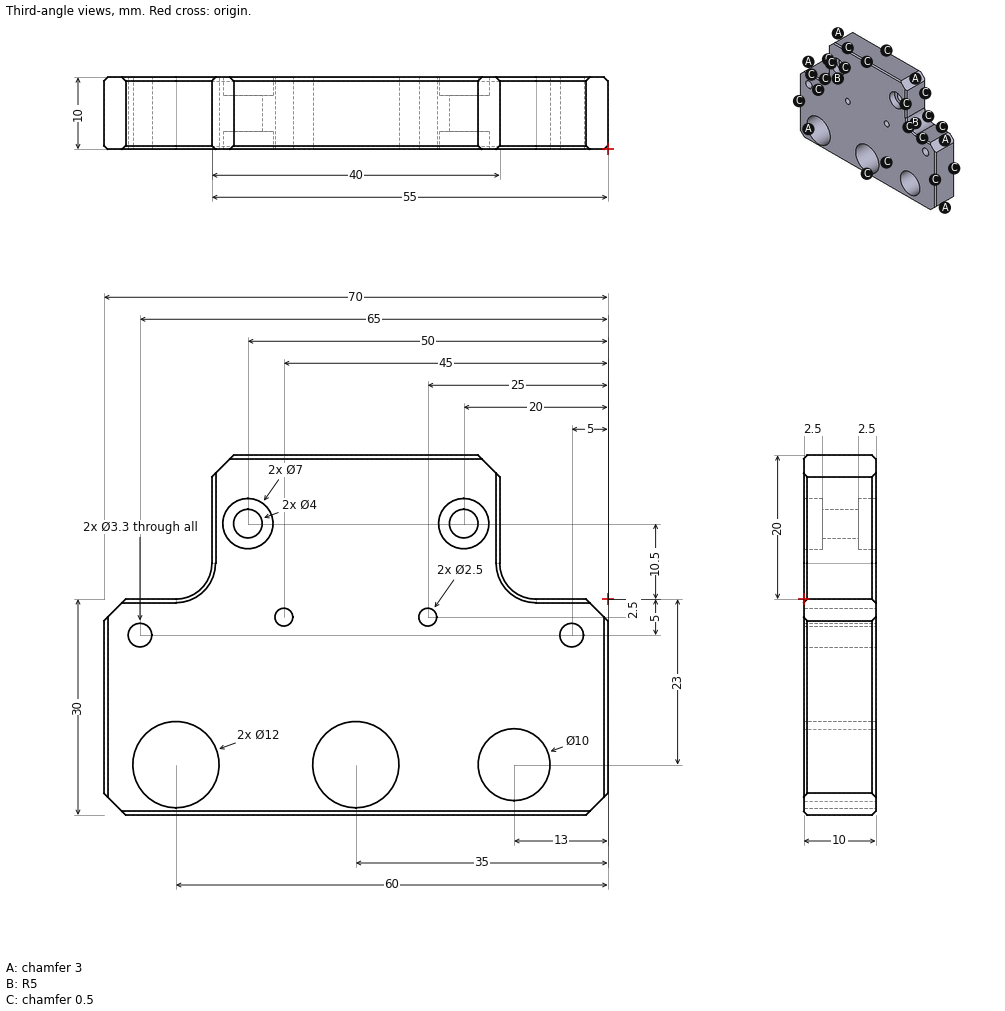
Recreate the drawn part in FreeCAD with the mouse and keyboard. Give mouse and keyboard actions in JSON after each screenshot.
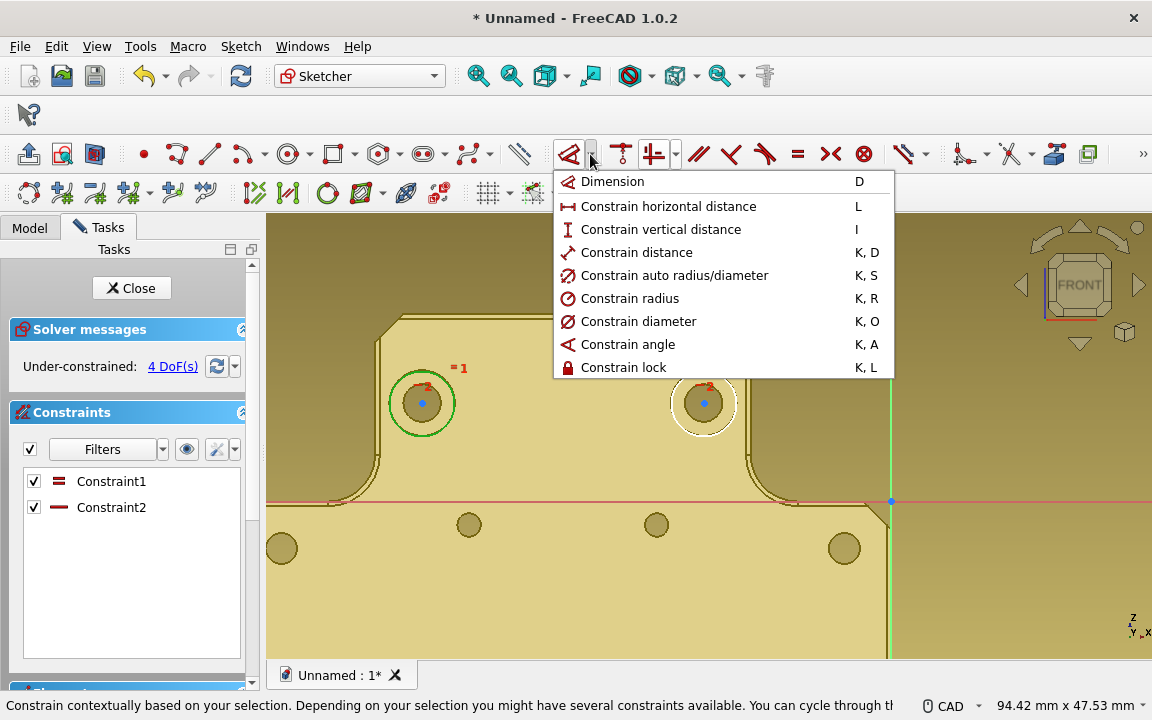
{"action": "left_click", "coordinate": [724, 322]}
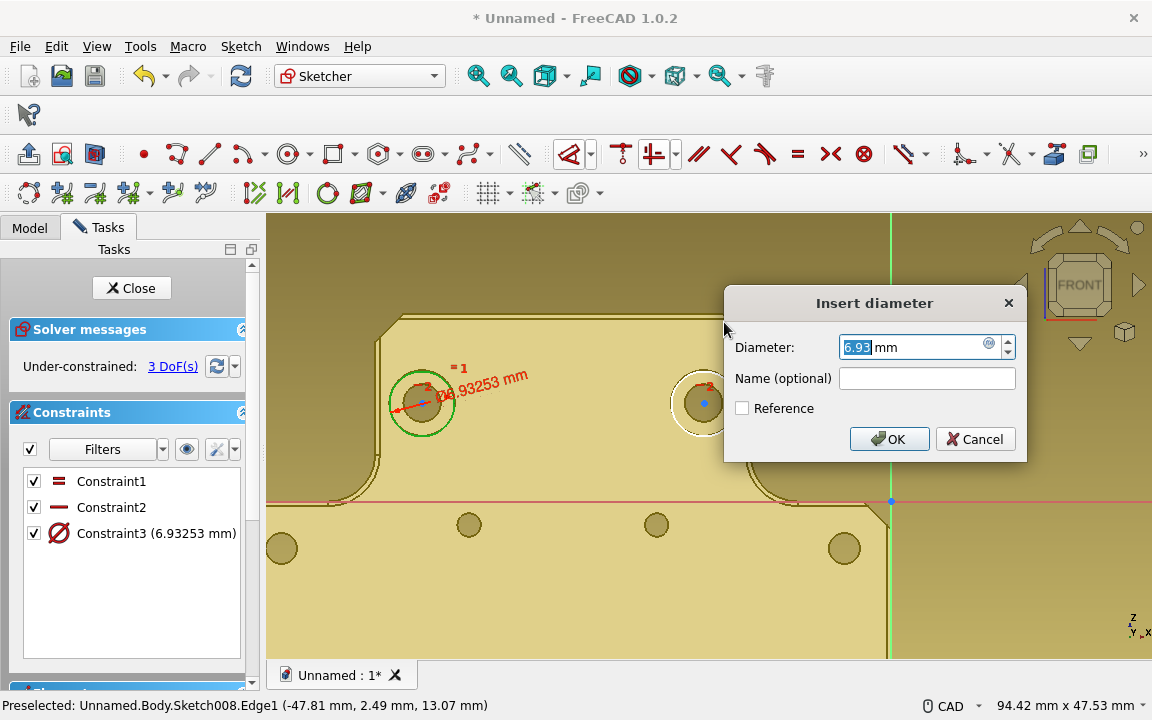
{"action": "type", "text": "7"}
{"action": "key", "text": "Return"}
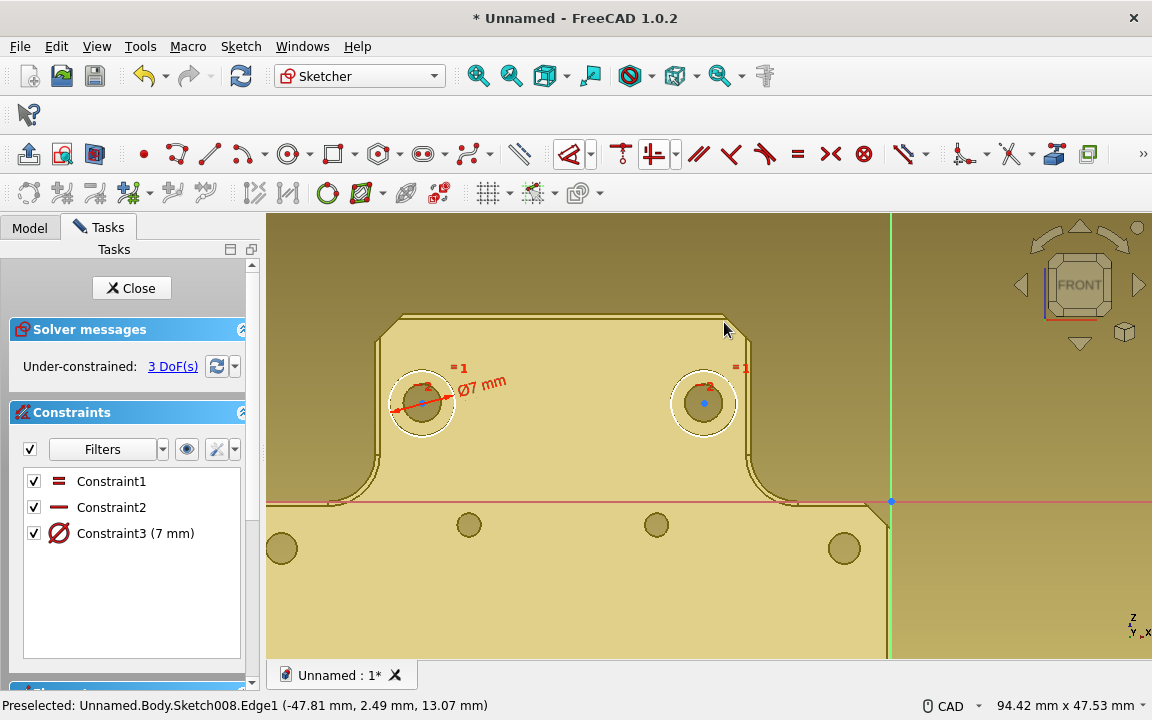
{"action": "left_click", "coordinate": [422, 404]}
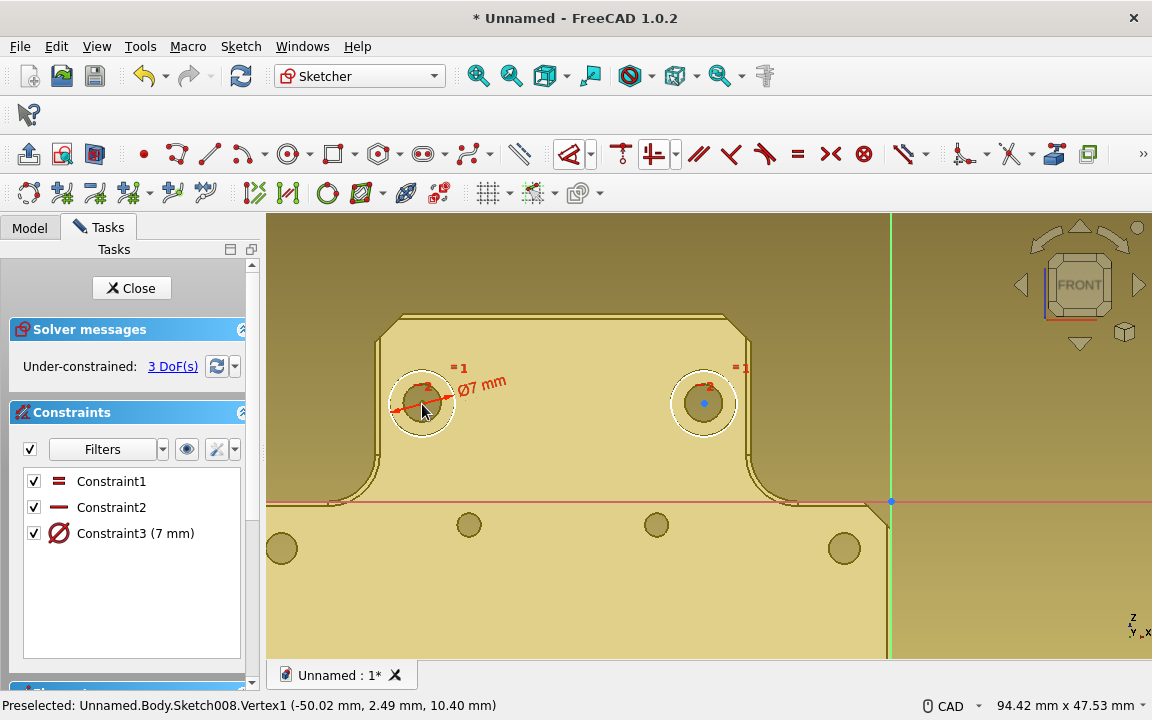
{"action": "left_click", "coordinate": [590, 154]}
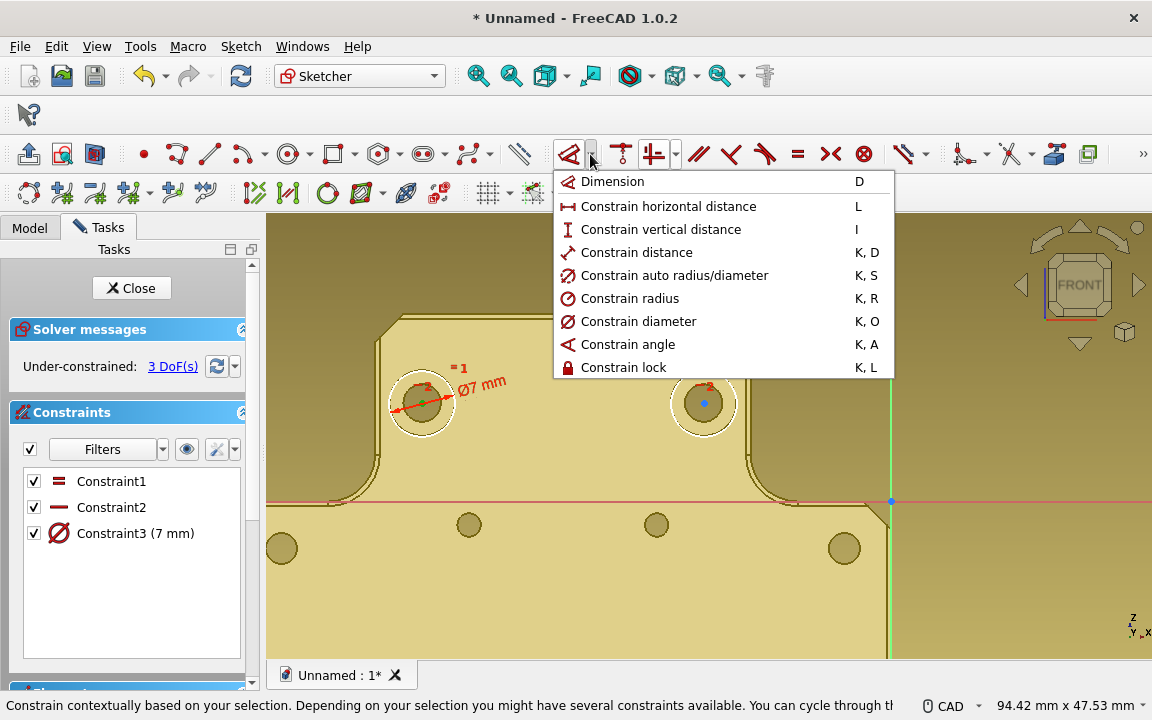
{"action": "left_click", "coordinate": [724, 206]}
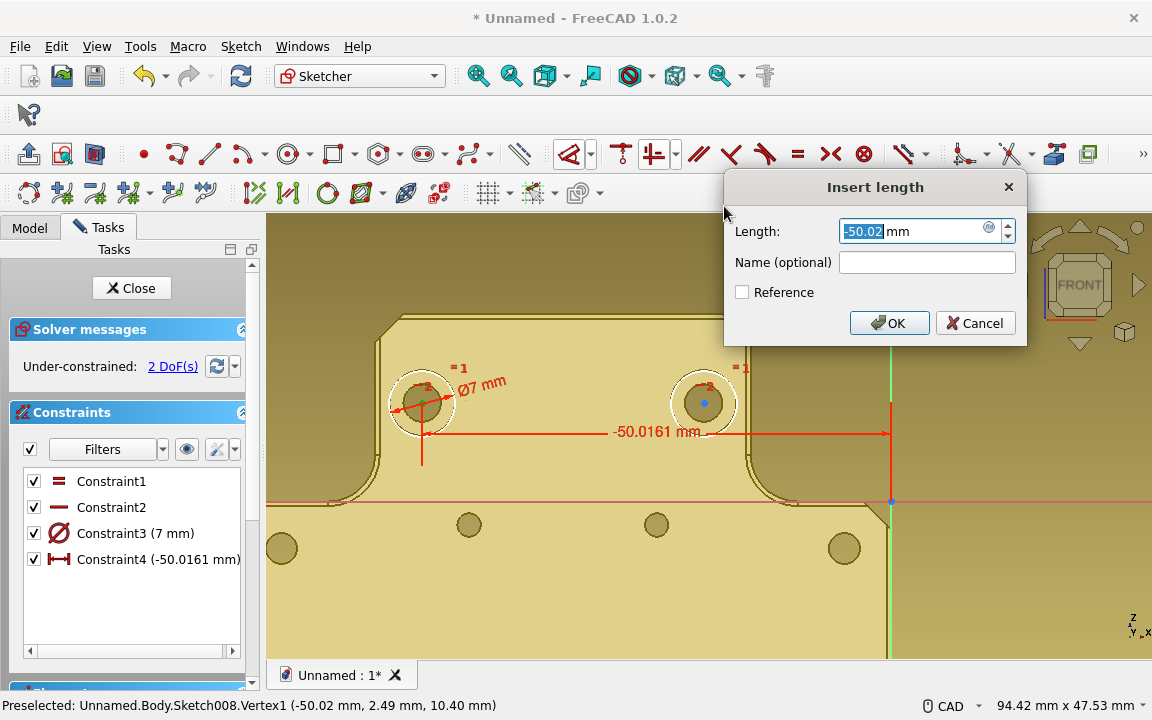
{"action": "type", "text": "-50"}
{"action": "key", "text": "Return"}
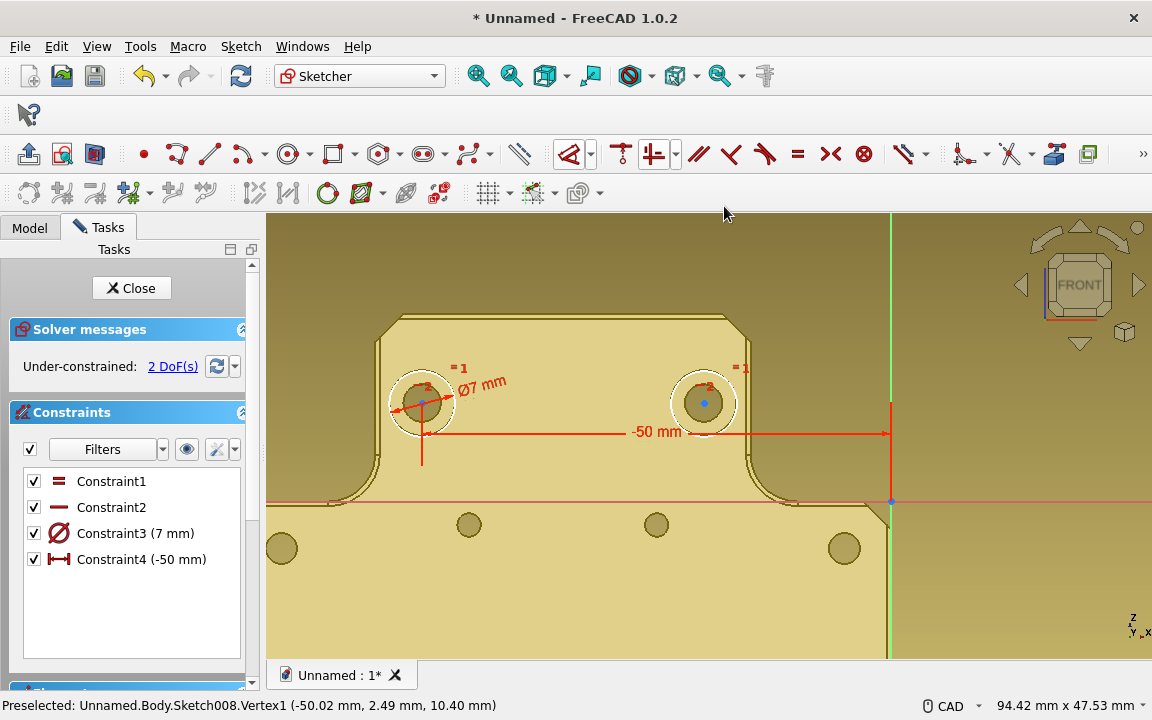
{"action": "left_click", "coordinate": [704, 404]}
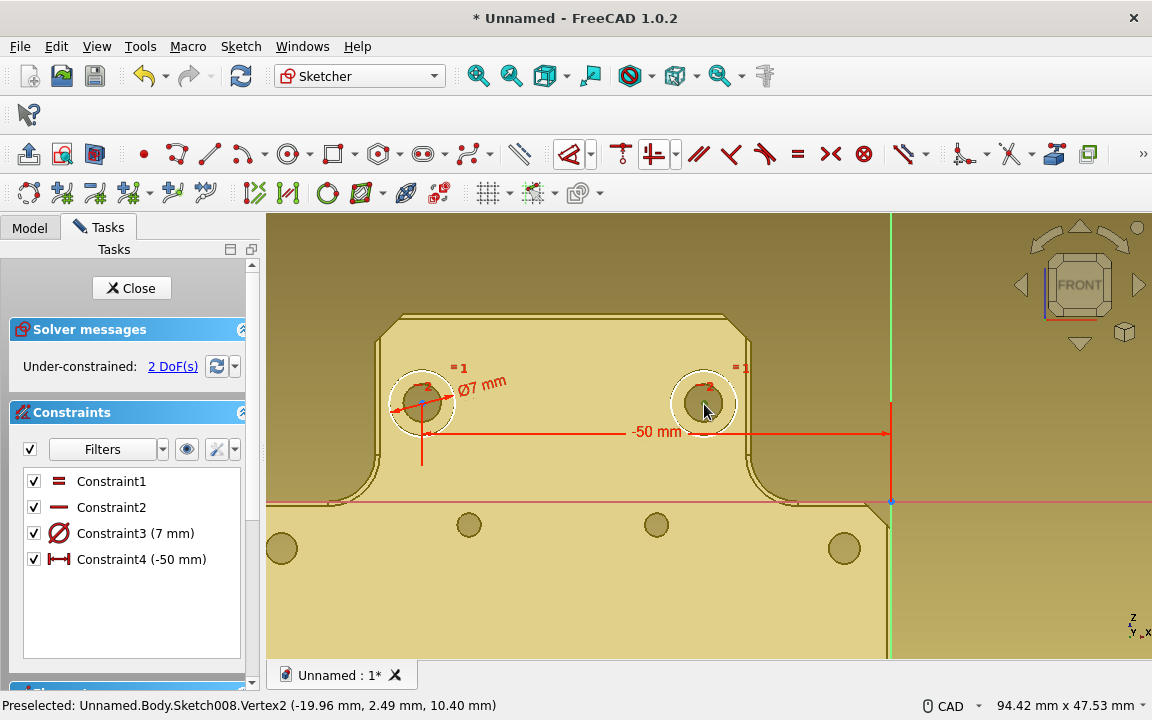
{"action": "left_click", "coordinate": [590, 154]}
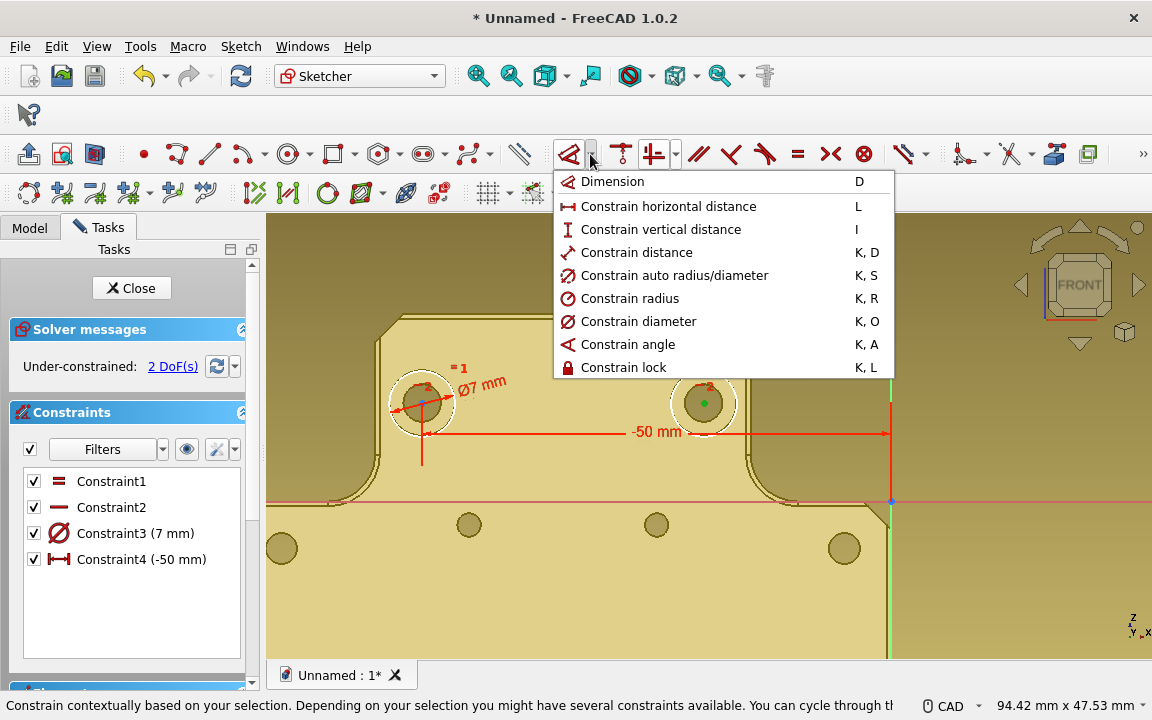
{"action": "left_click", "coordinate": [724, 206]}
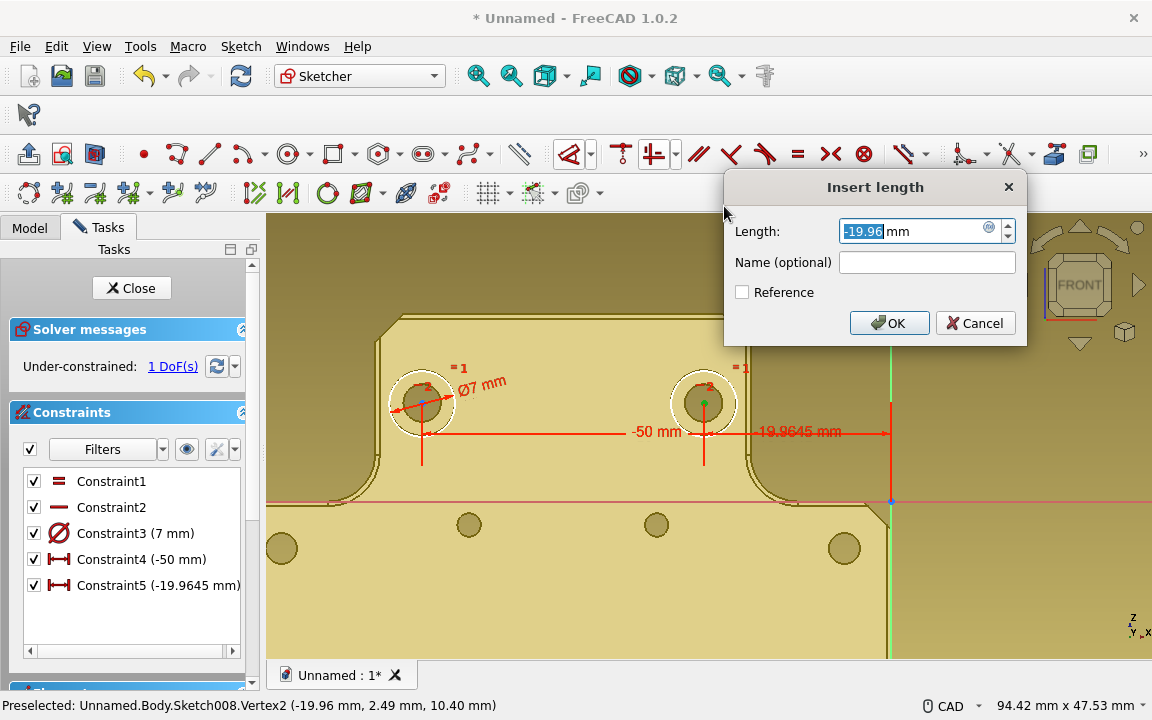
{"action": "type", "text": "-20"}
{"action": "key", "text": "Return"}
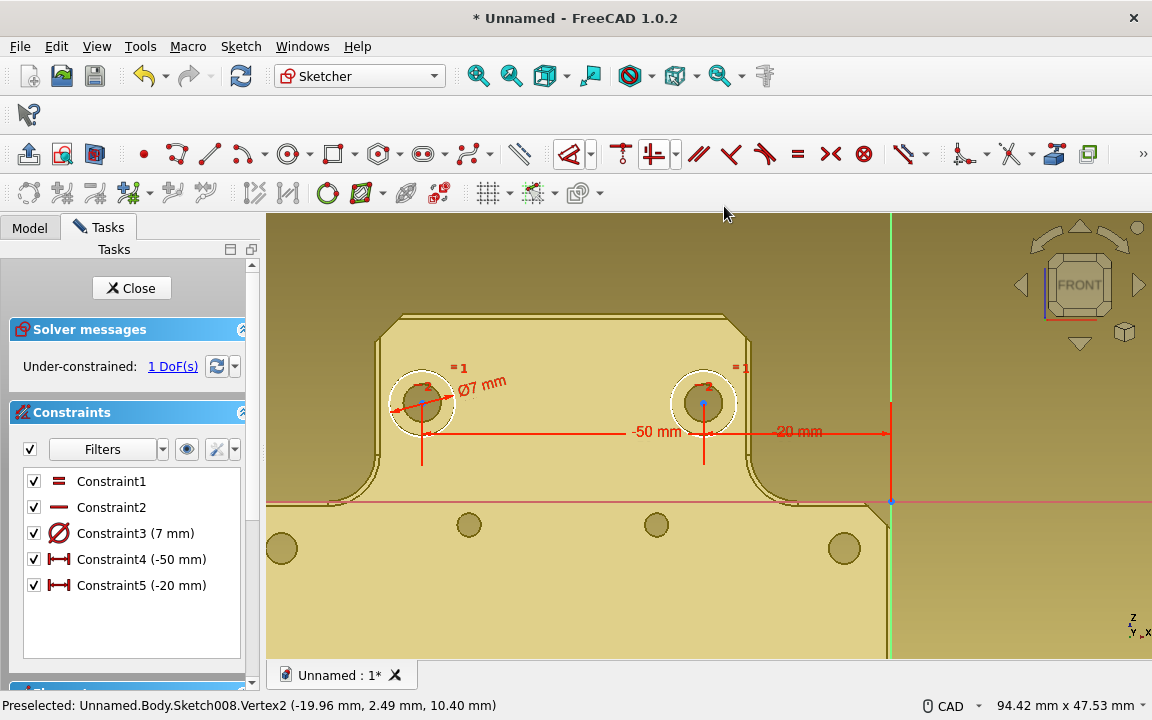
{"action": "left_click", "coordinate": [422, 404]}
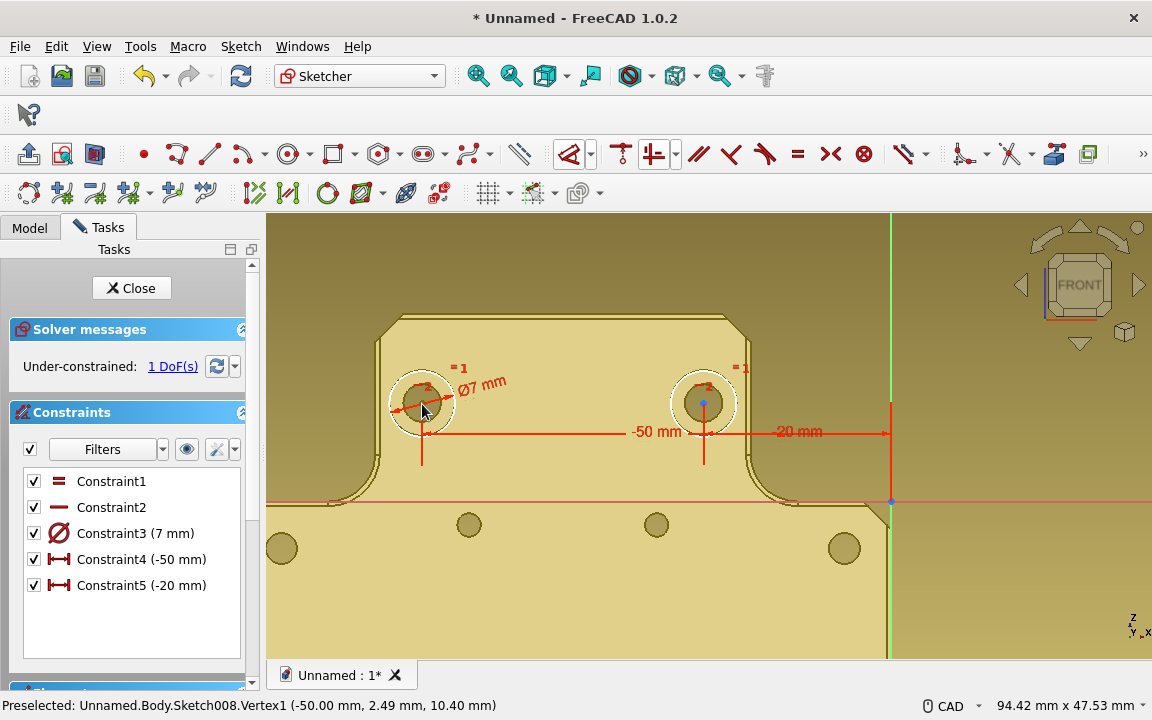
{"action": "key", "text": "i"}